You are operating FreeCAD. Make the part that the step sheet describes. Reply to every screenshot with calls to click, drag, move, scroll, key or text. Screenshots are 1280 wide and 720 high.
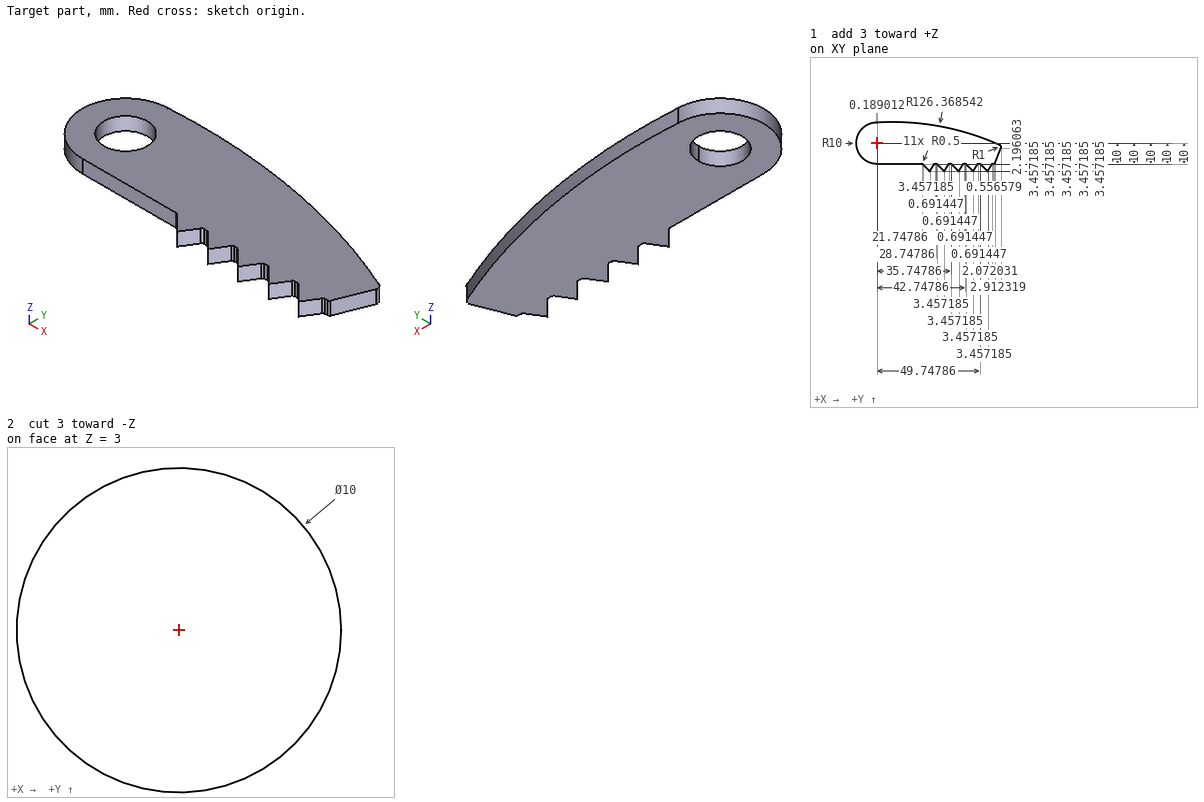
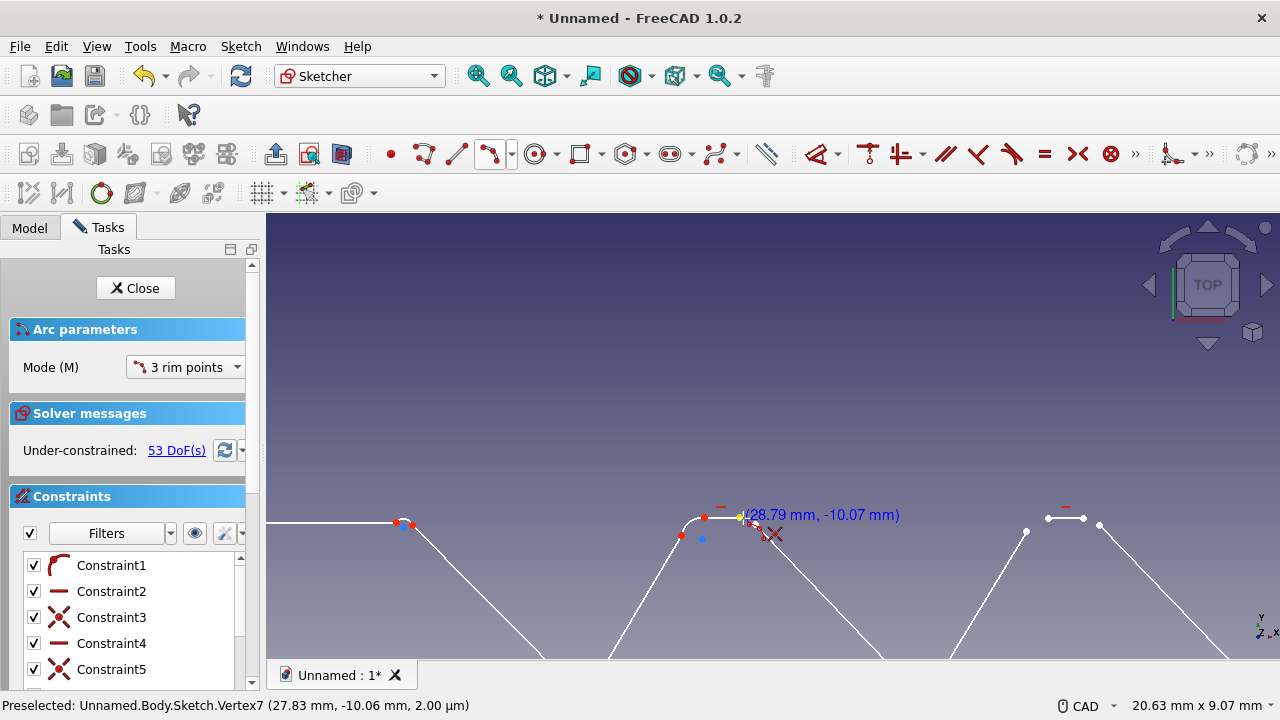
click(739, 518)
click(756, 525)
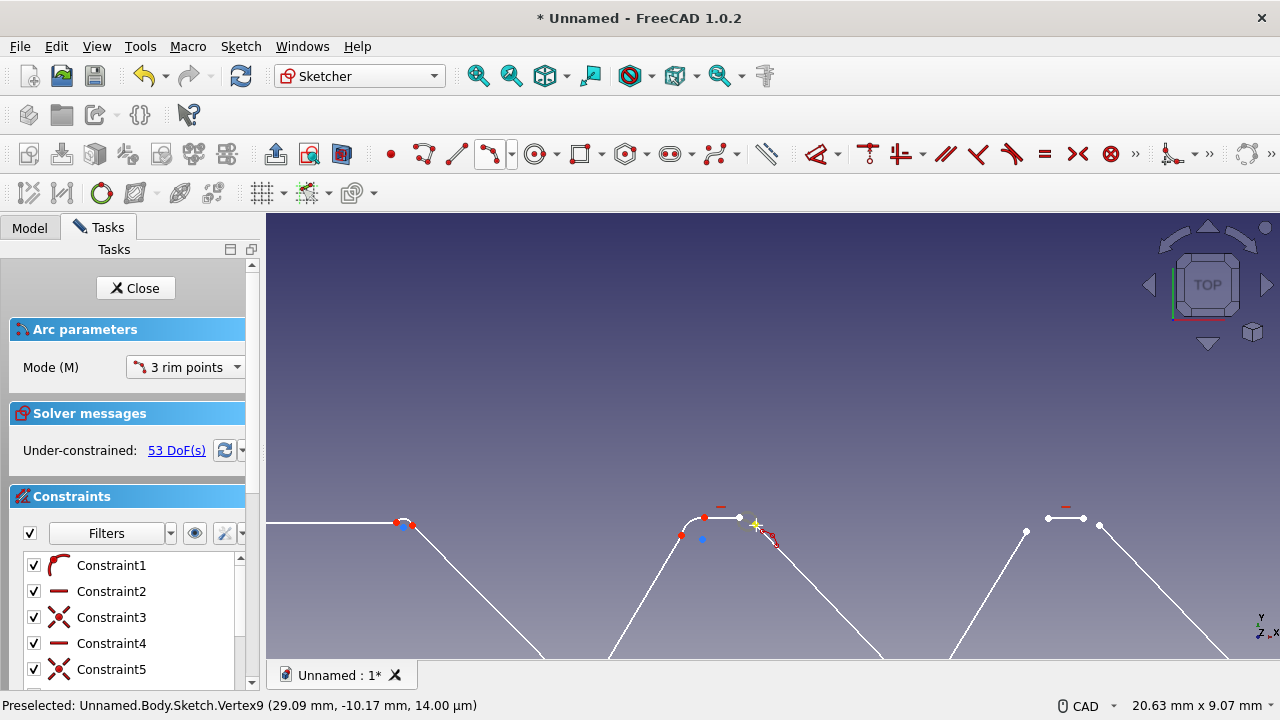
scroll(748, 519, up, 11)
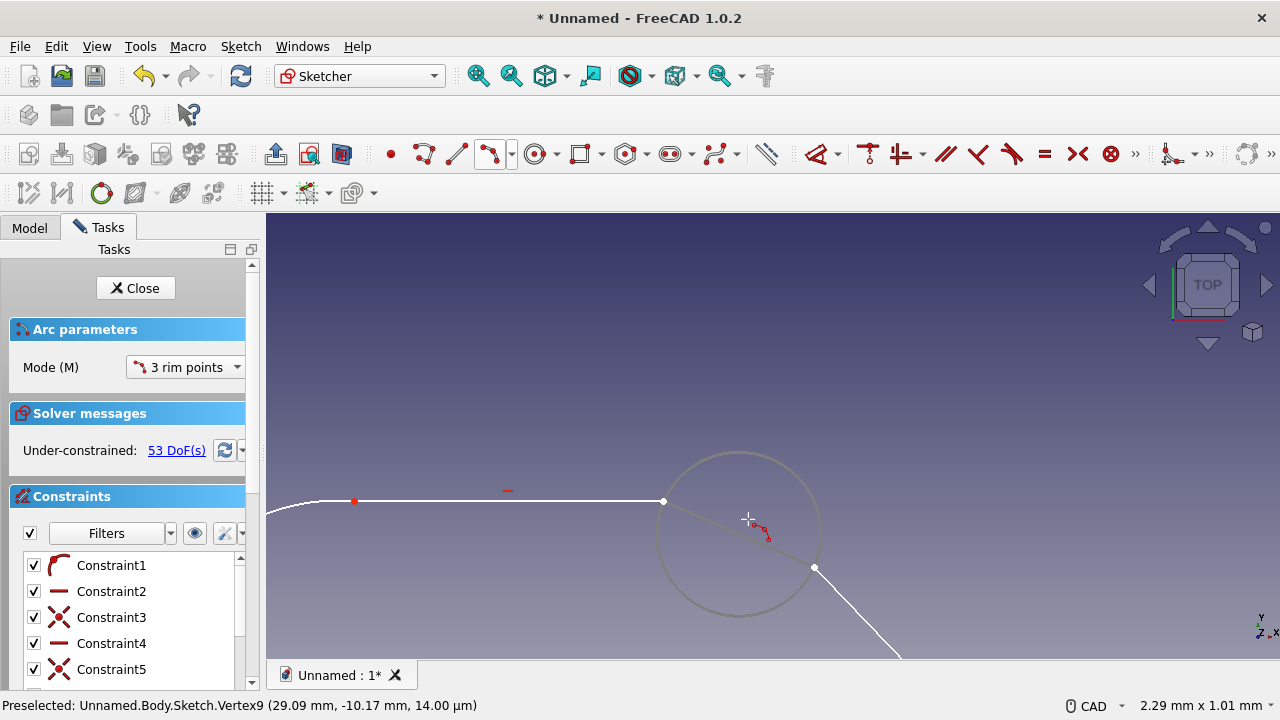
click(746, 511)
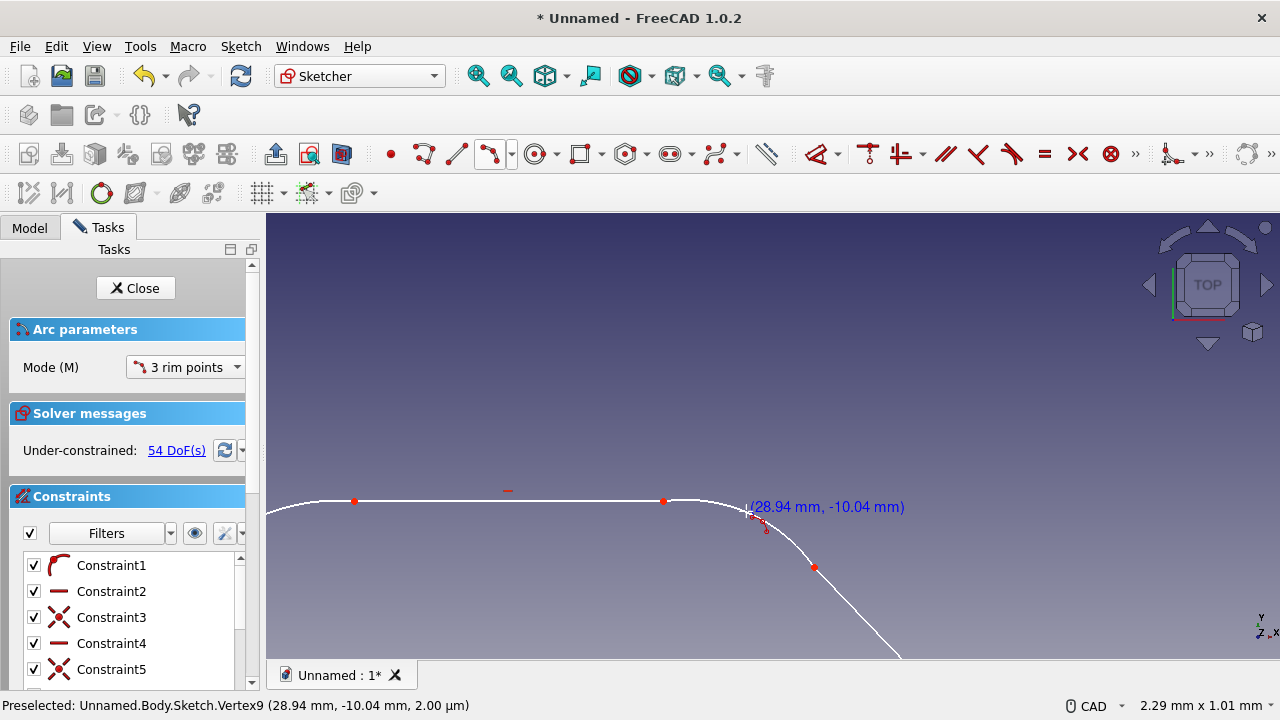
scroll(704, 436, down, 15)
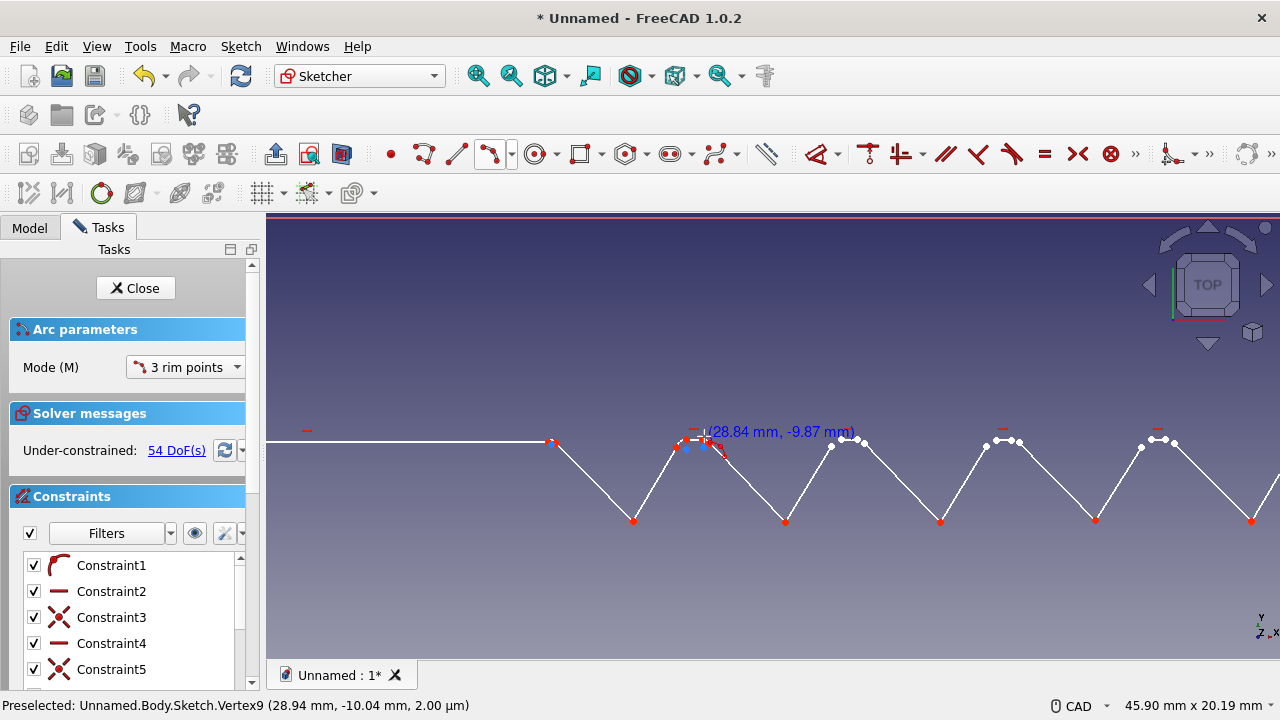
scroll(754, 539, down, 5)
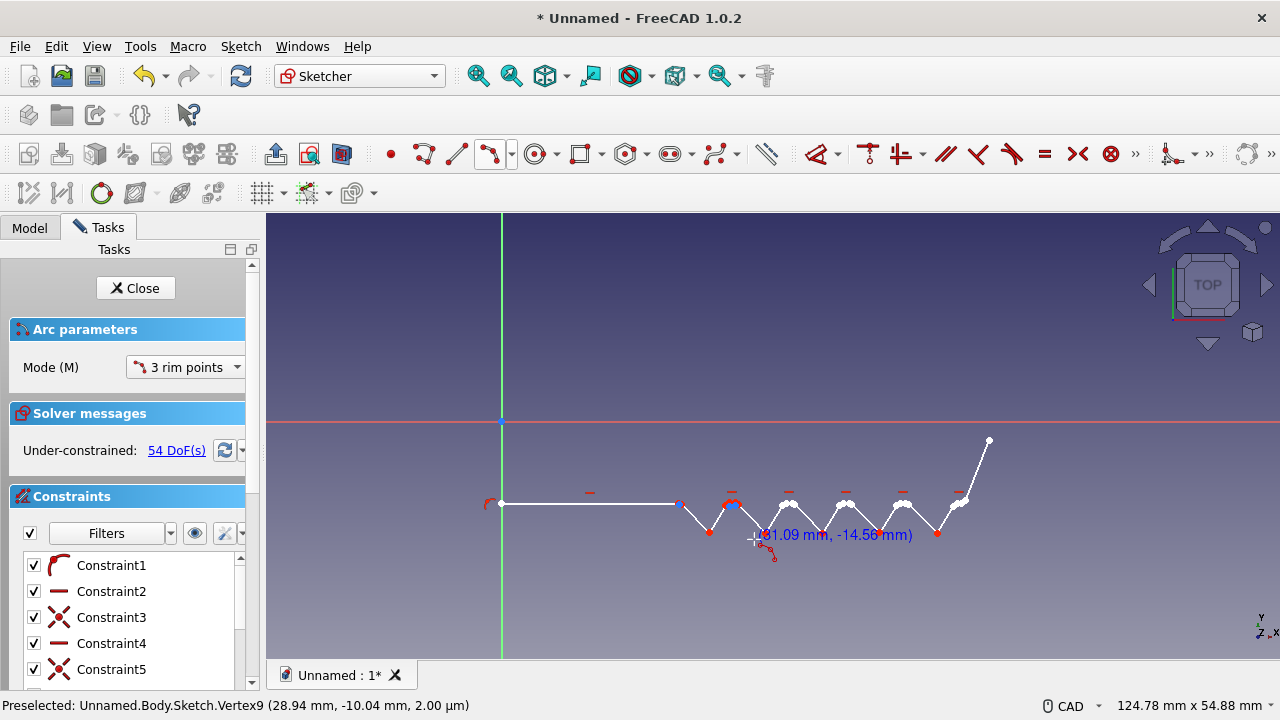
scroll(783, 505, up, 7)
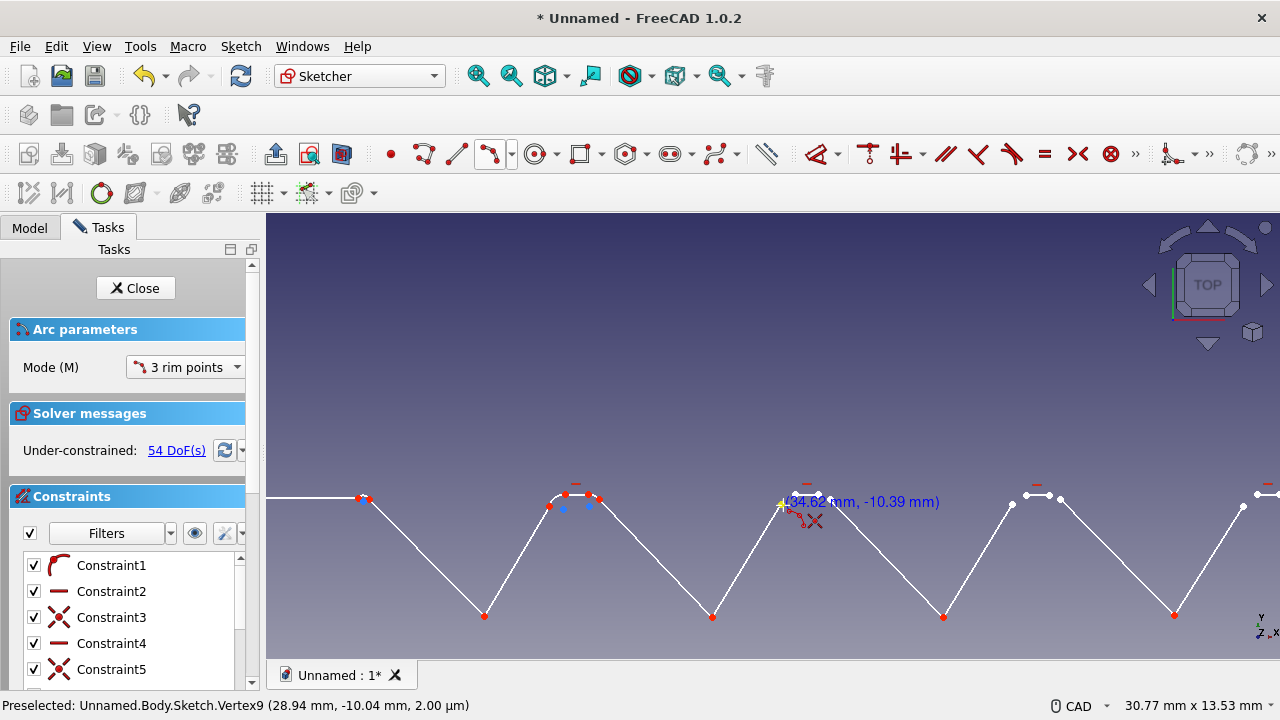
click(781, 504)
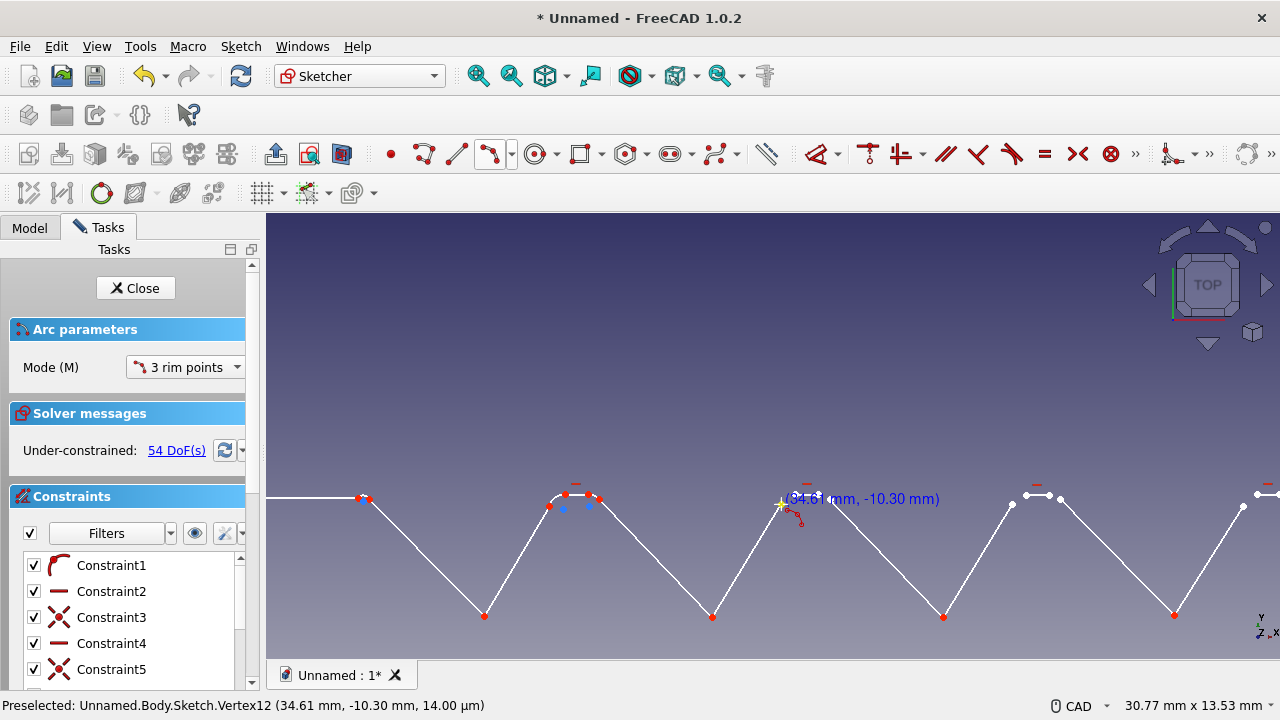
scroll(796, 494, up, 2)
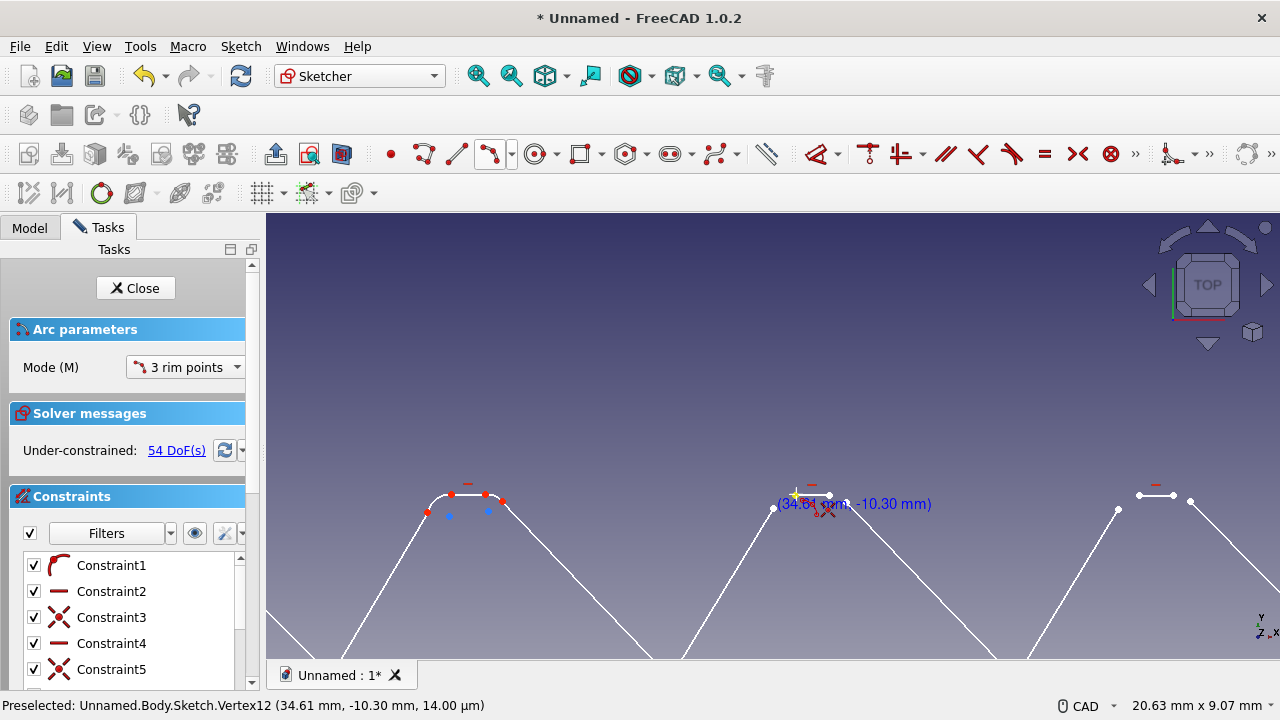
click(795, 495)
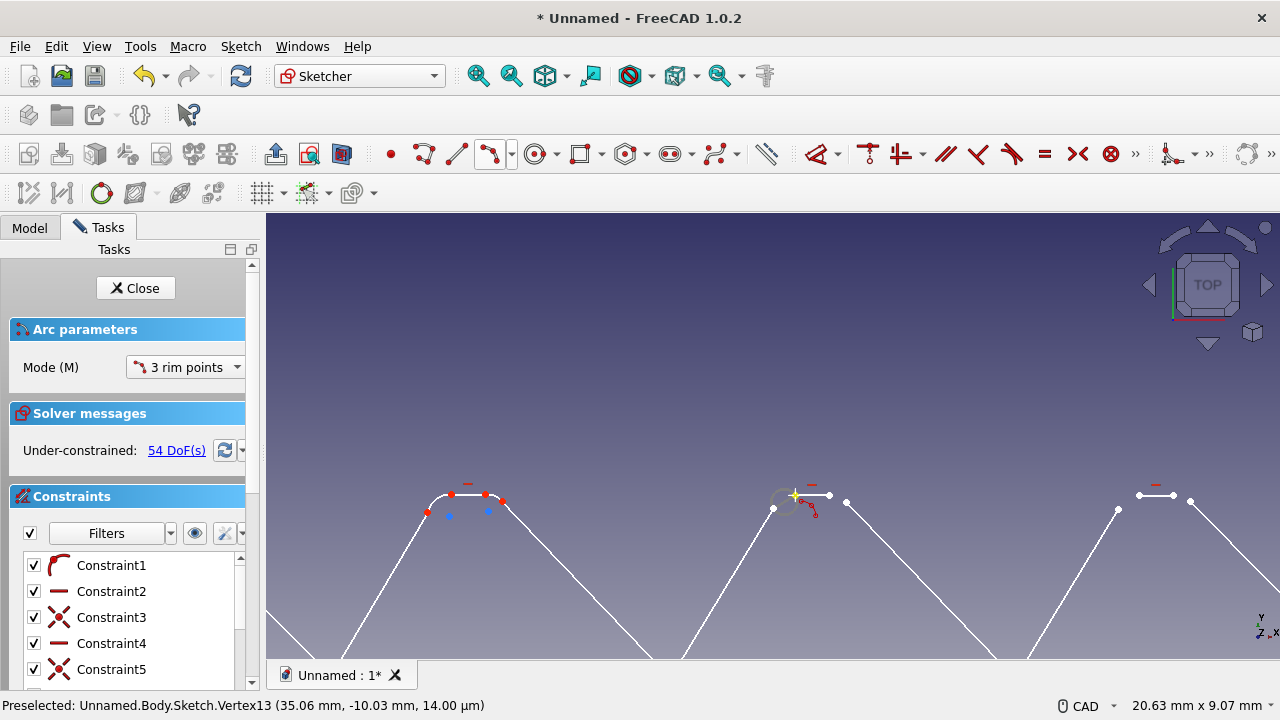
scroll(784, 497, up, 9)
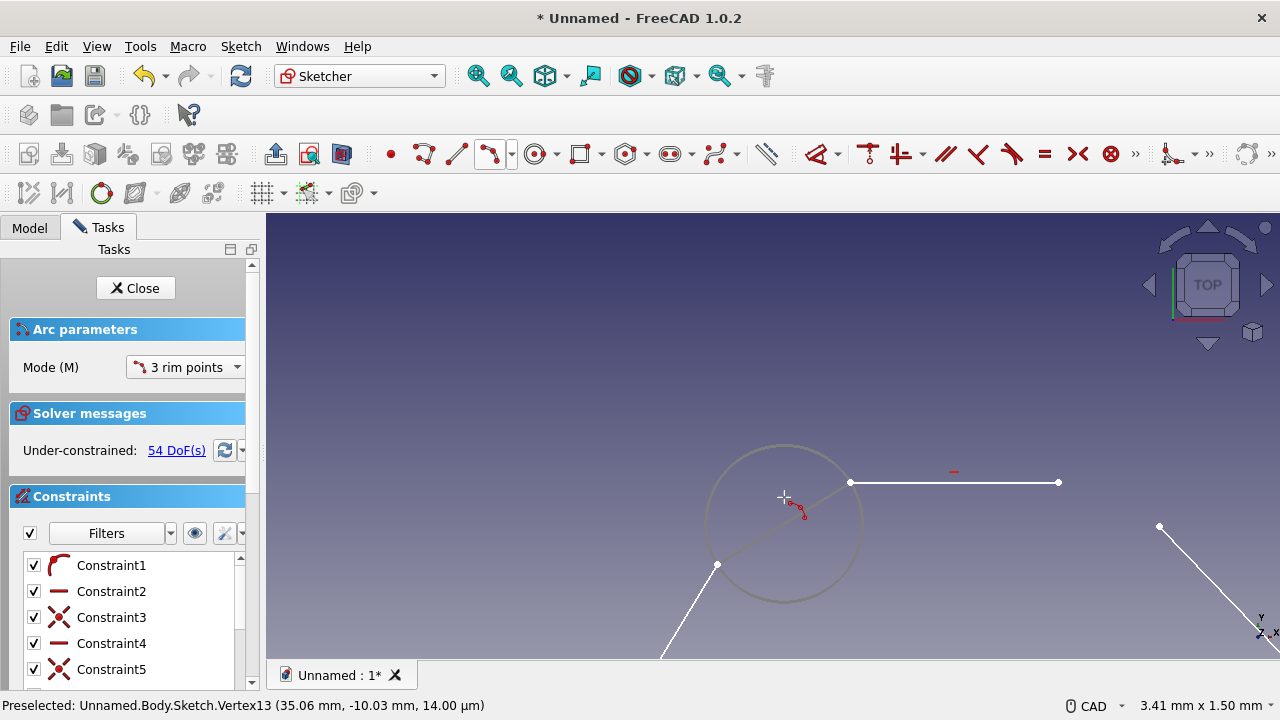
click(778, 494)